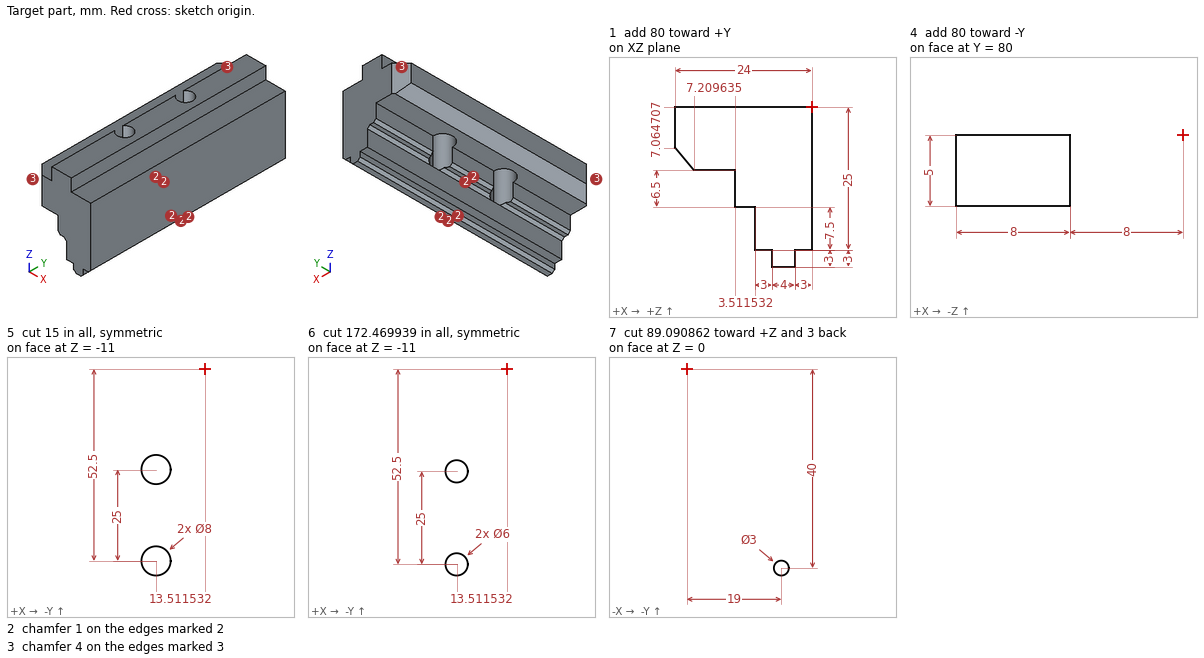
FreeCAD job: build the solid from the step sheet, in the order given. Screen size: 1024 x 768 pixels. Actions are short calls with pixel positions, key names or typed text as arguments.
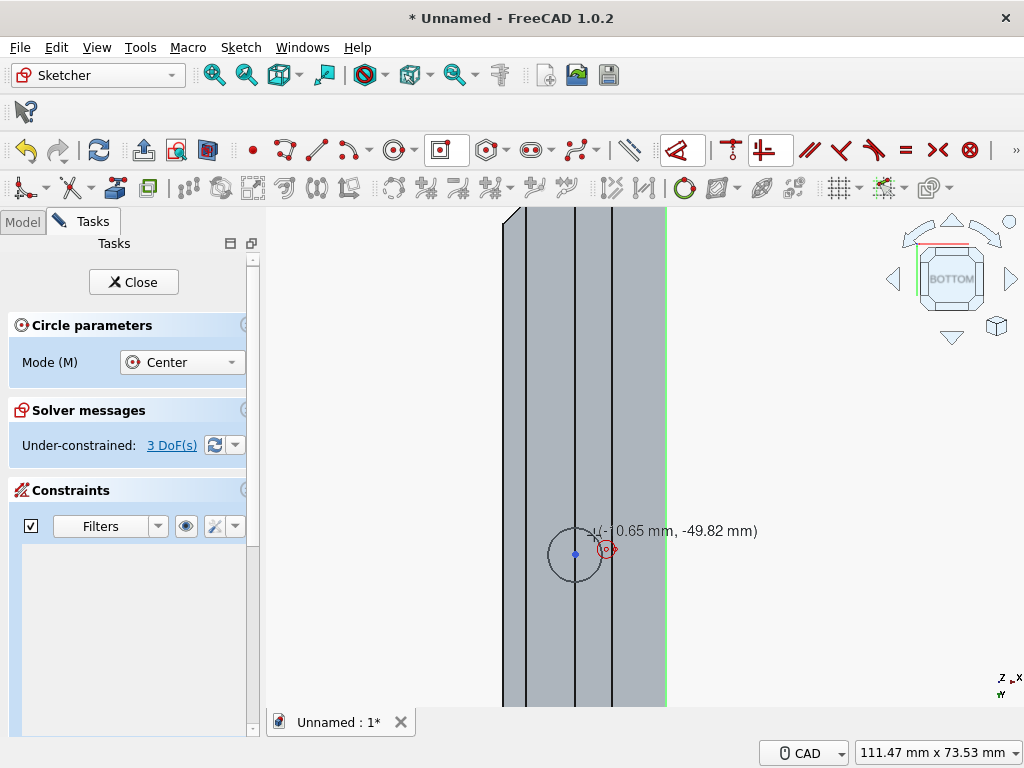
click(575, 384)
click(594, 365)
key(Escape)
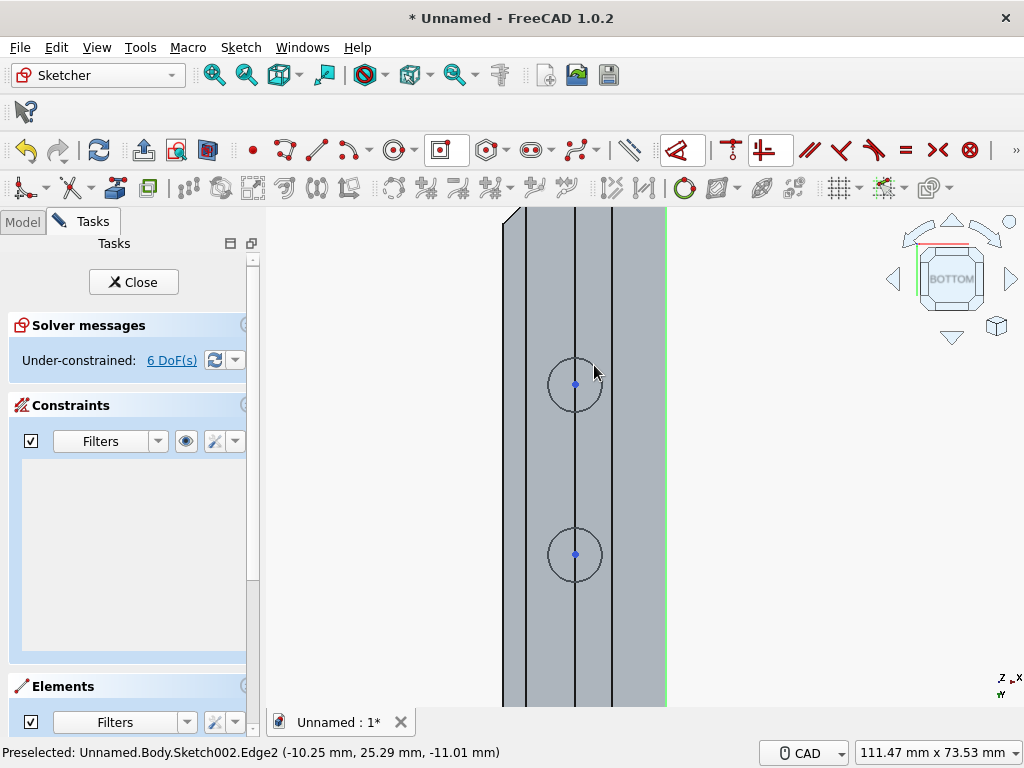
click(594, 536)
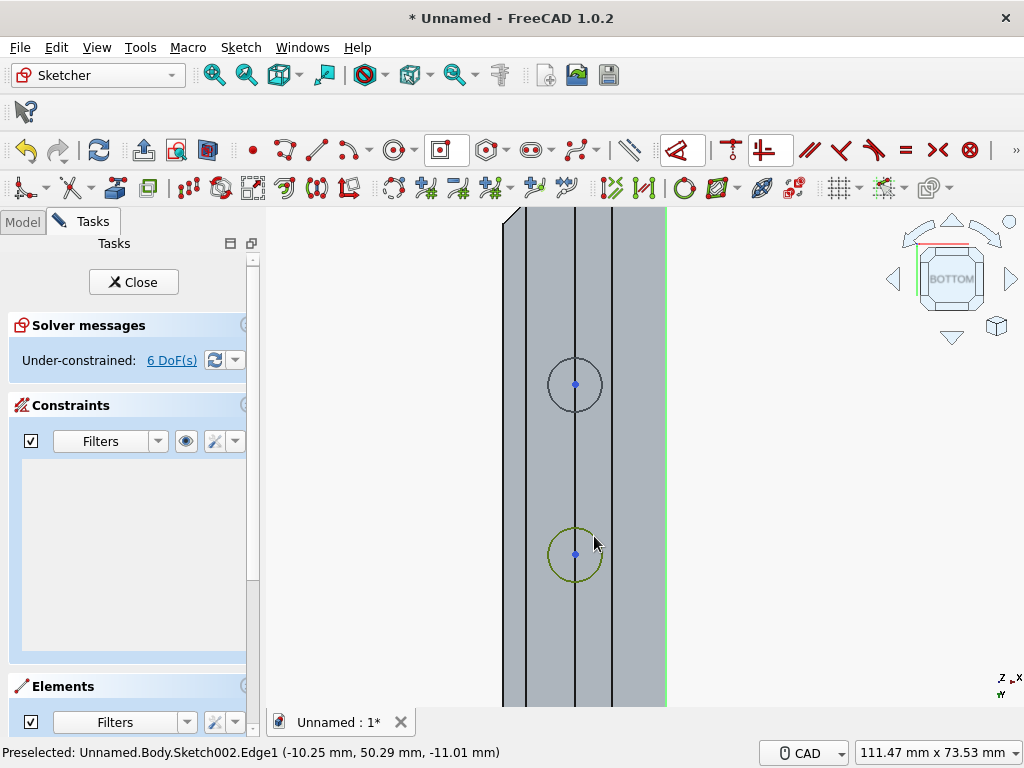
click(594, 366)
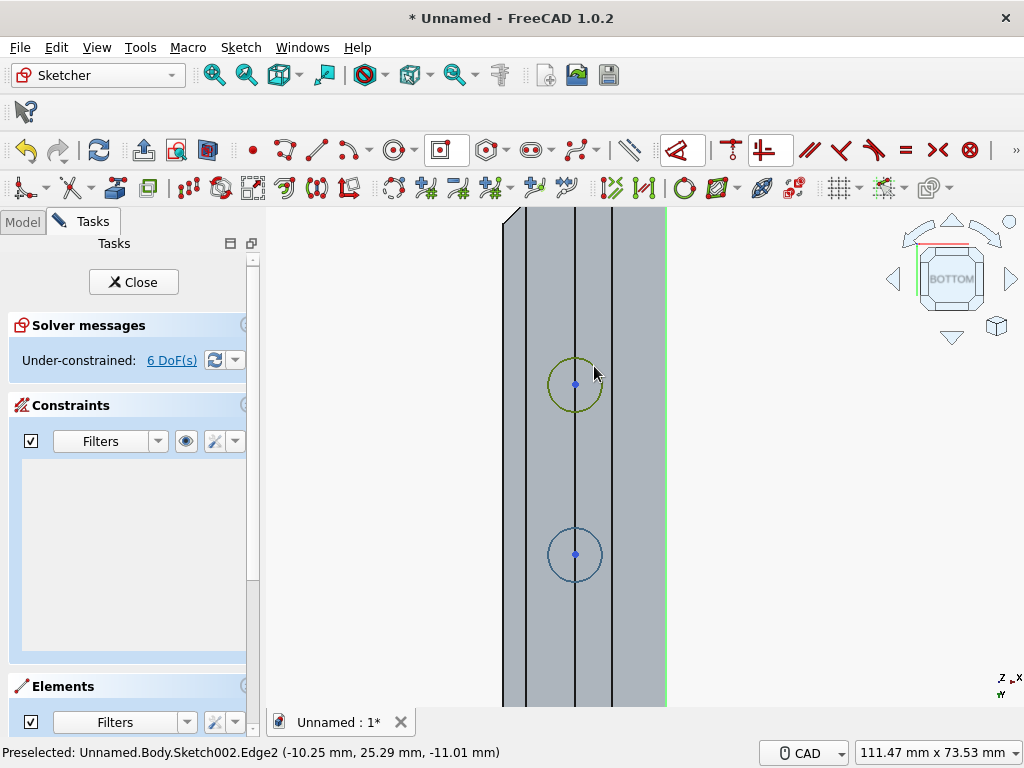
click(906, 150)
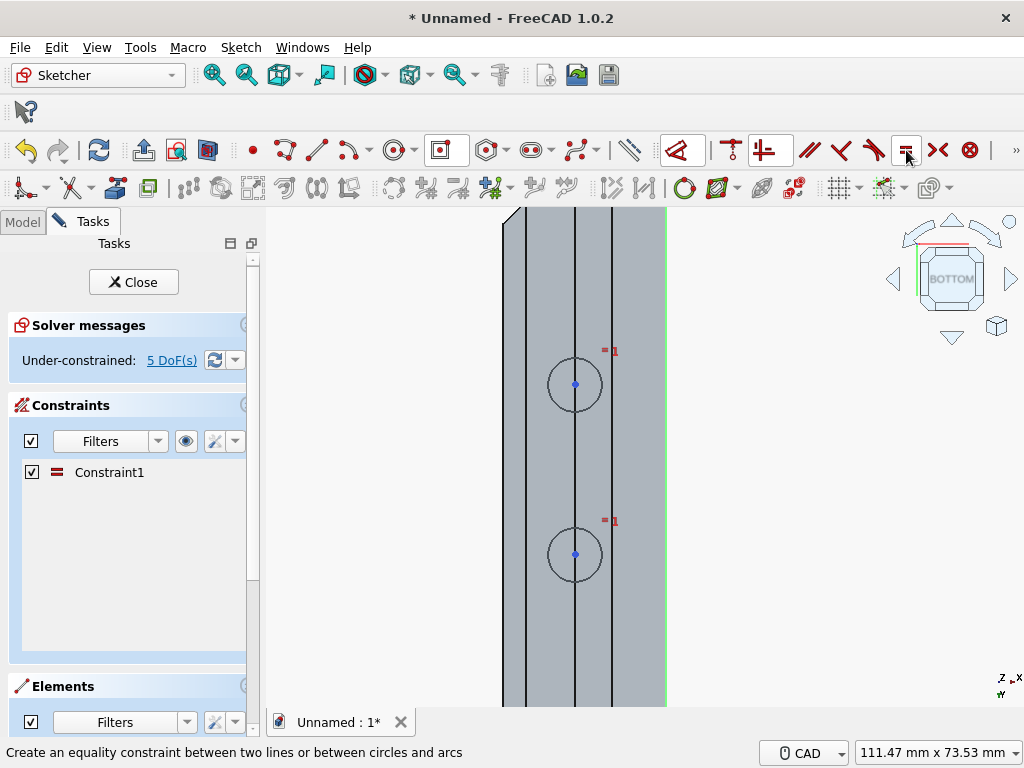
click(575, 555)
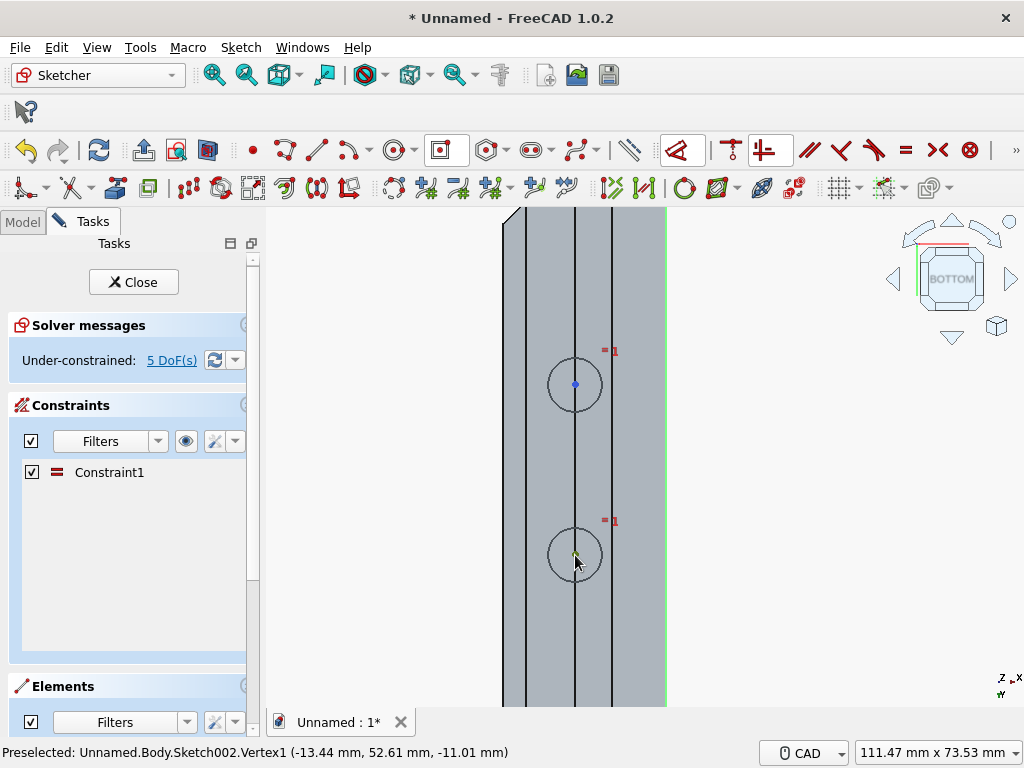
click(575, 385)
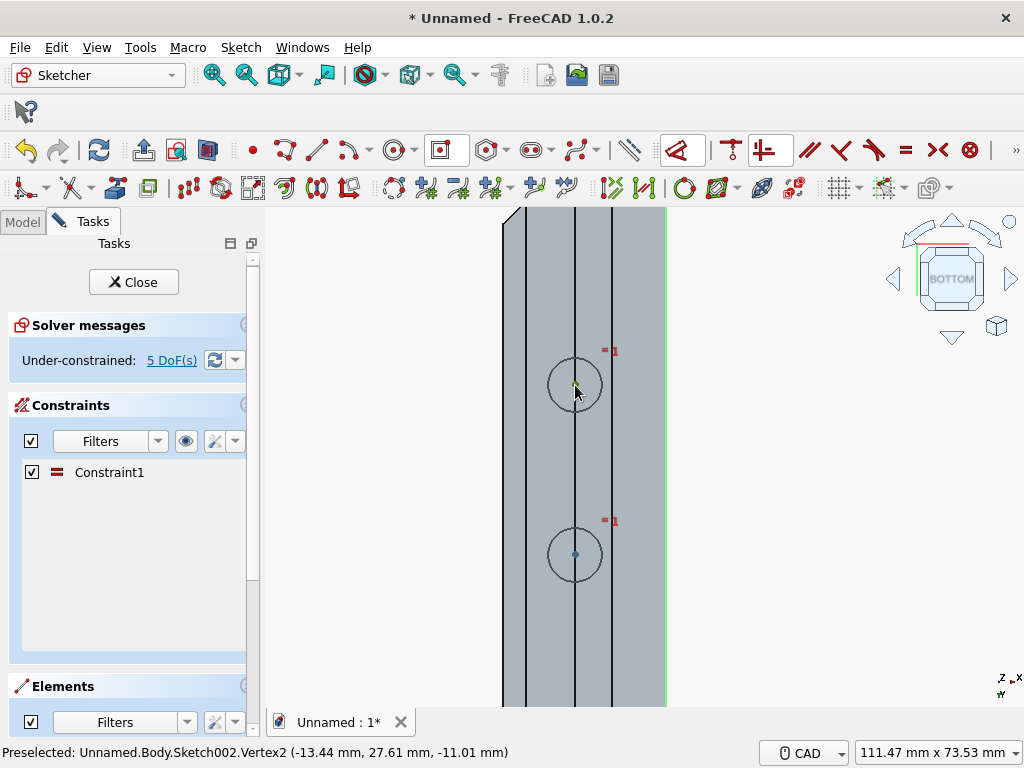
key(v)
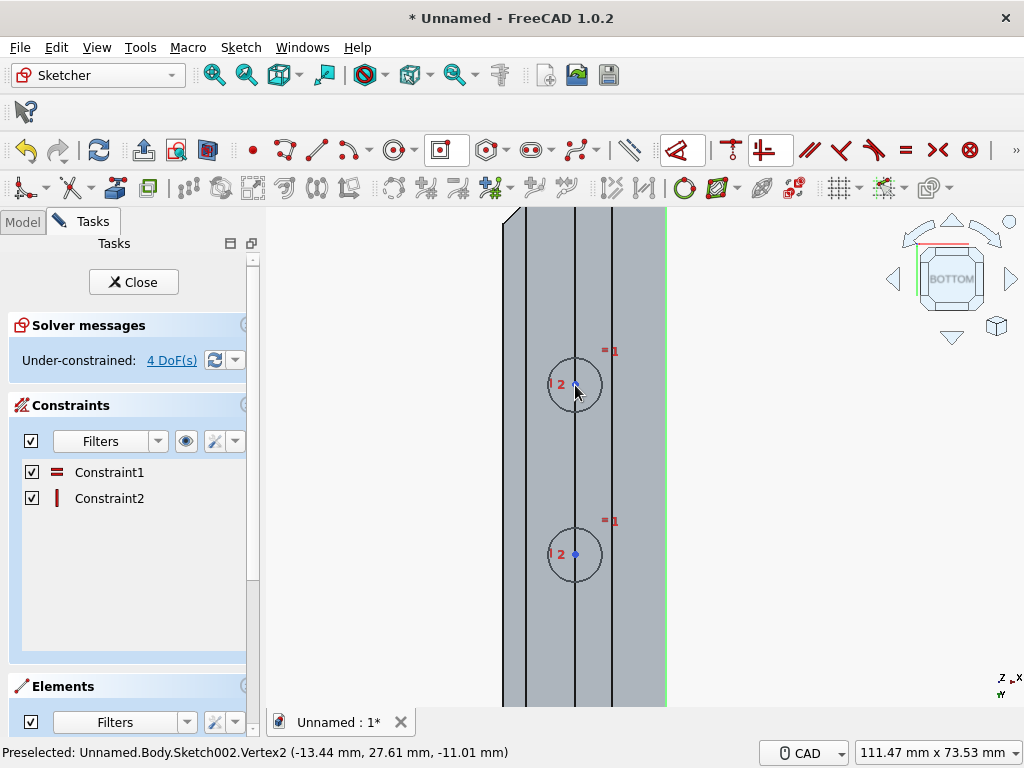
click(594, 536)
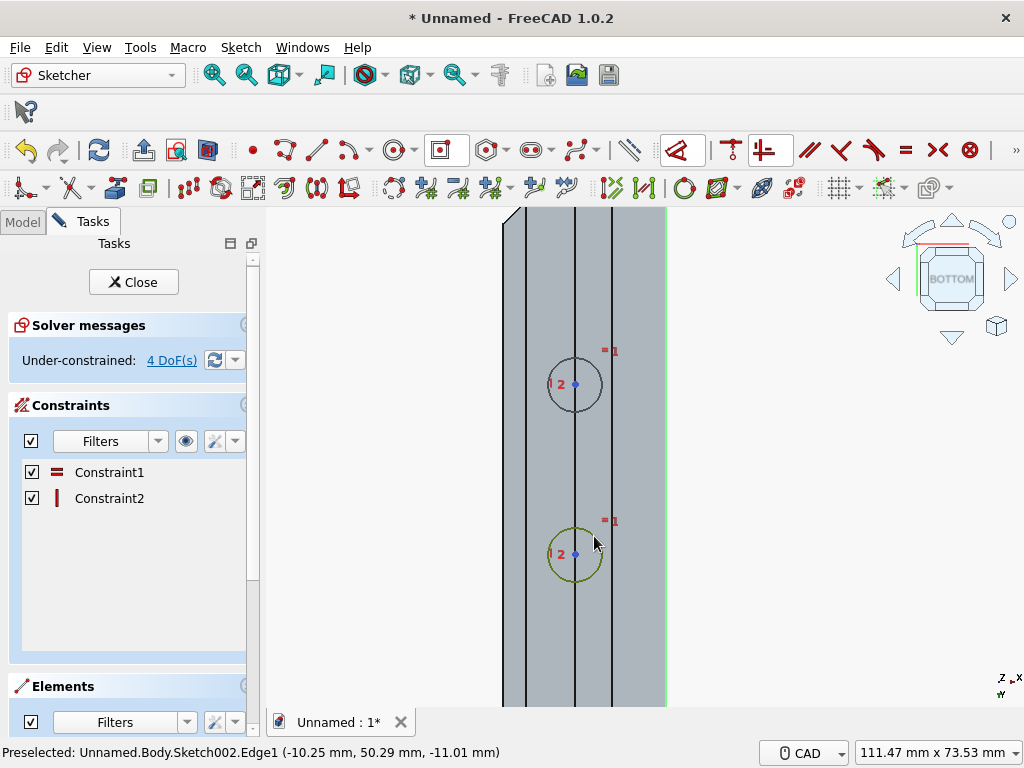
key(k)
key(o)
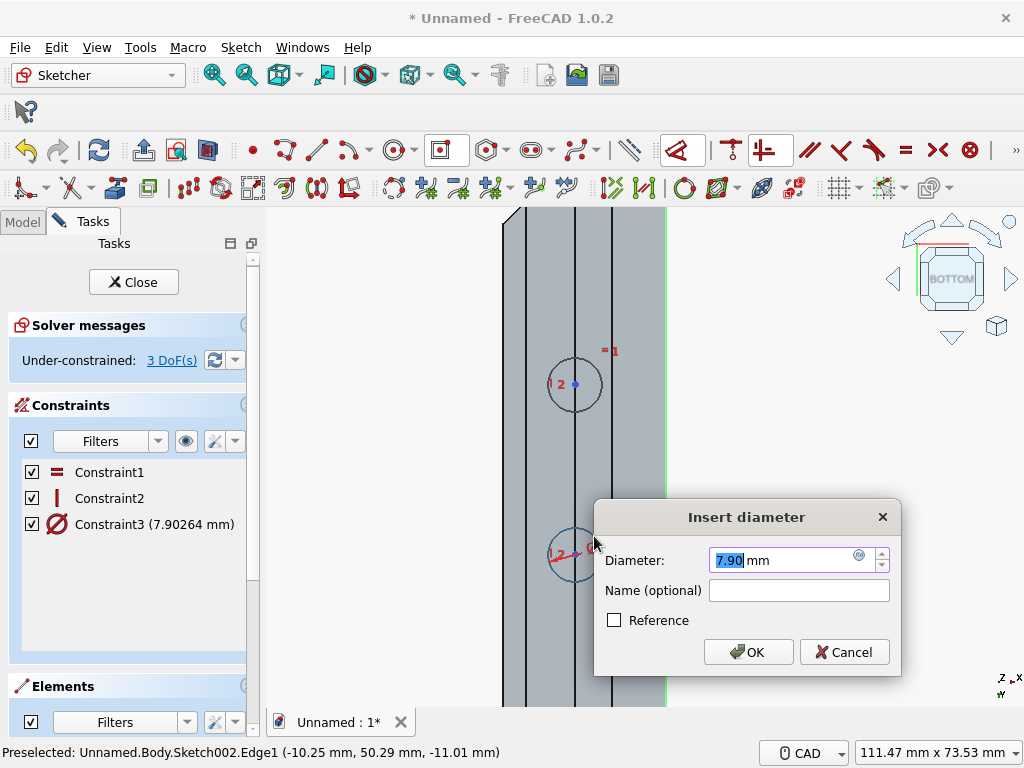
text(8)
key(Return)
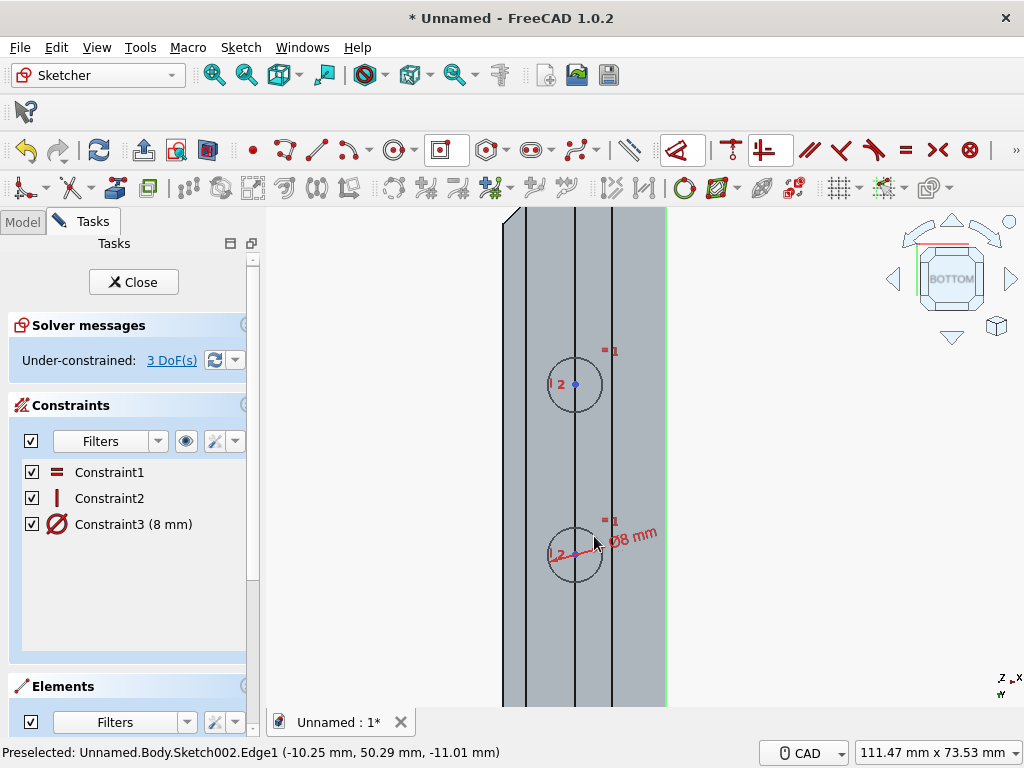
click(575, 555)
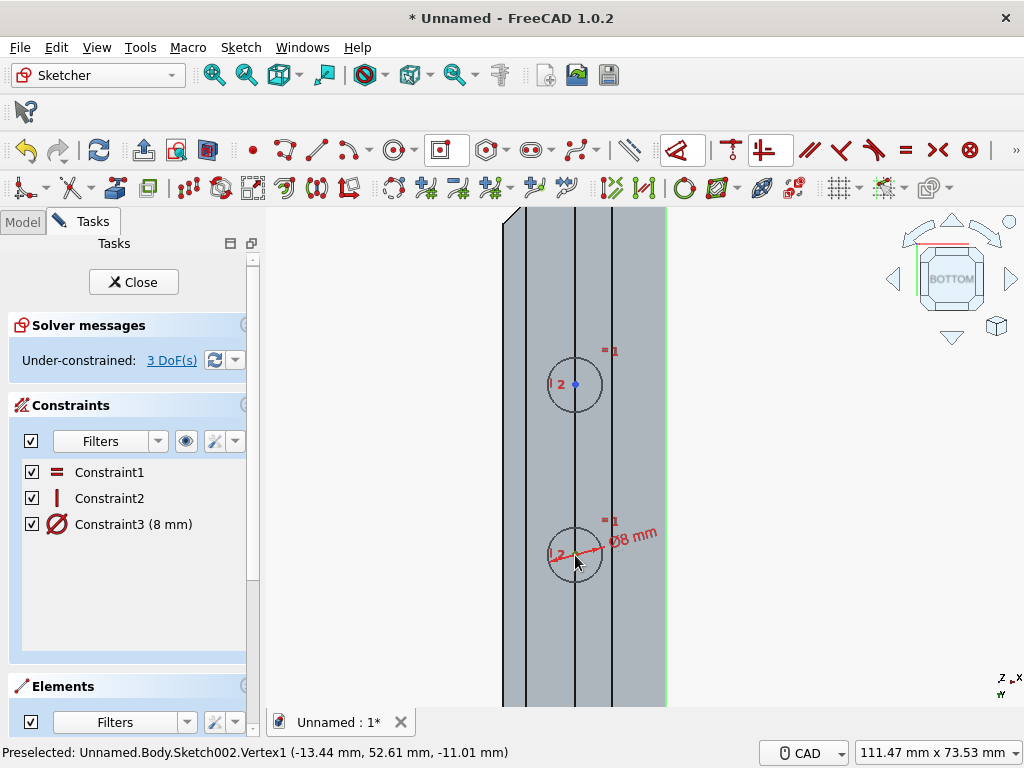
click(575, 385)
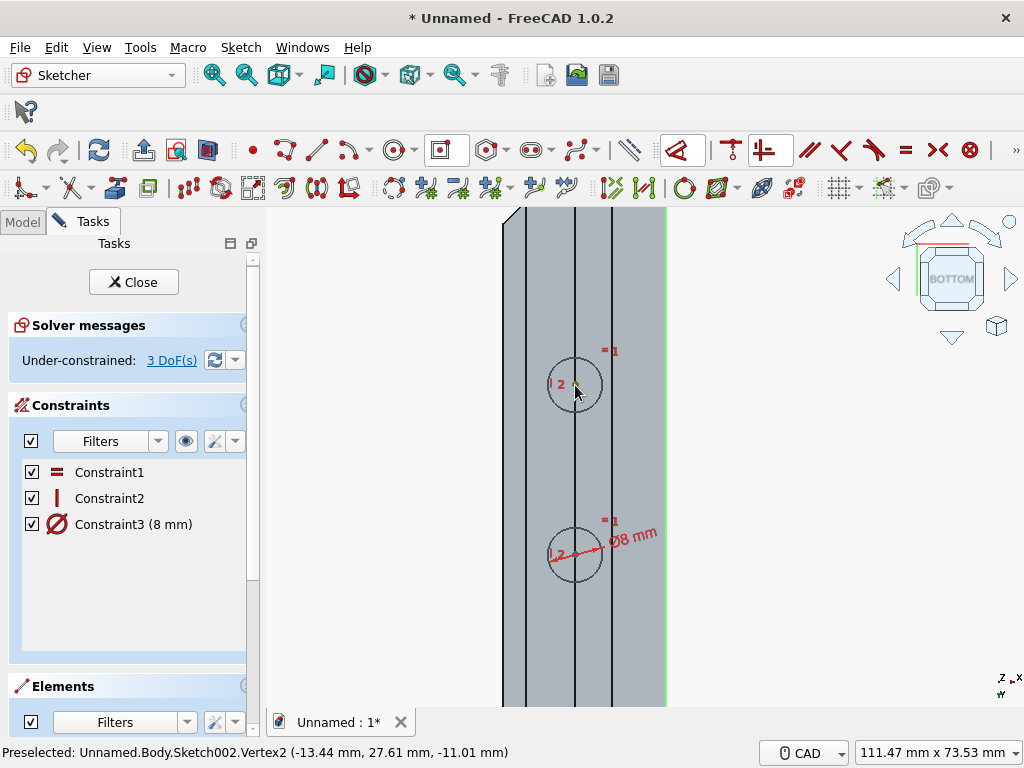
key(i)